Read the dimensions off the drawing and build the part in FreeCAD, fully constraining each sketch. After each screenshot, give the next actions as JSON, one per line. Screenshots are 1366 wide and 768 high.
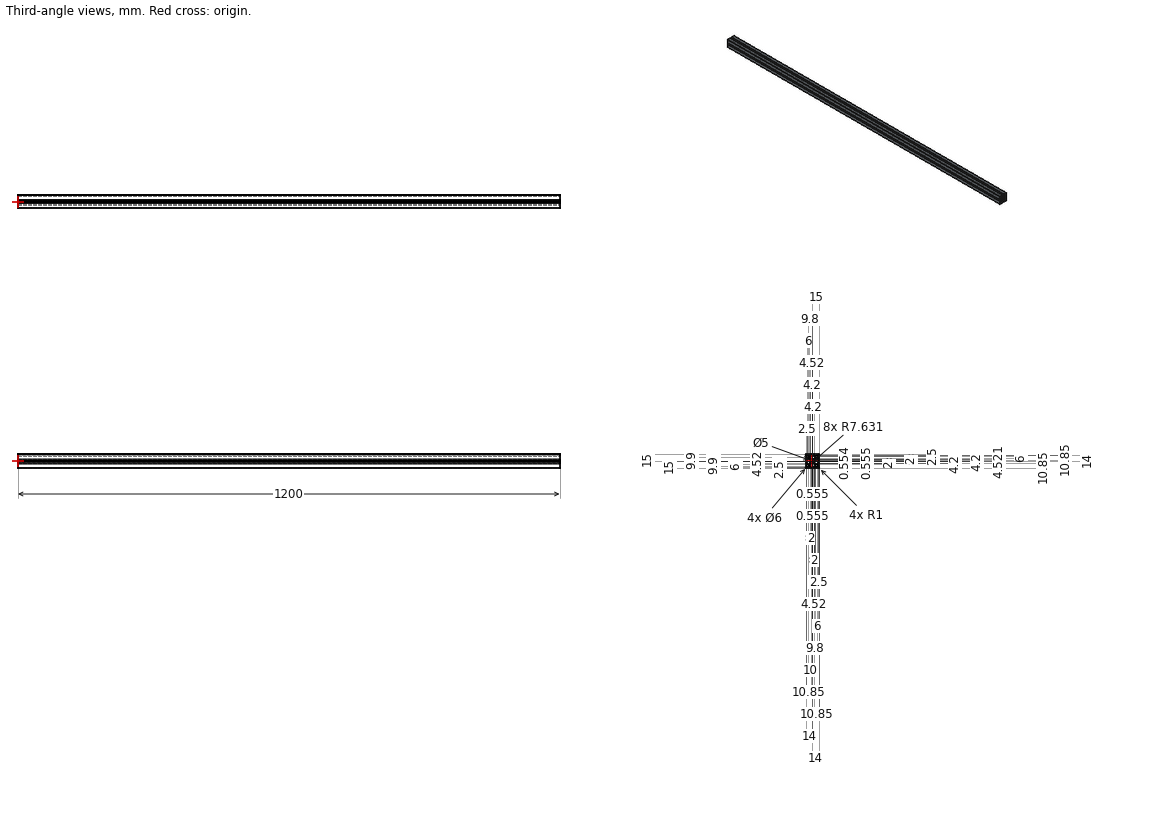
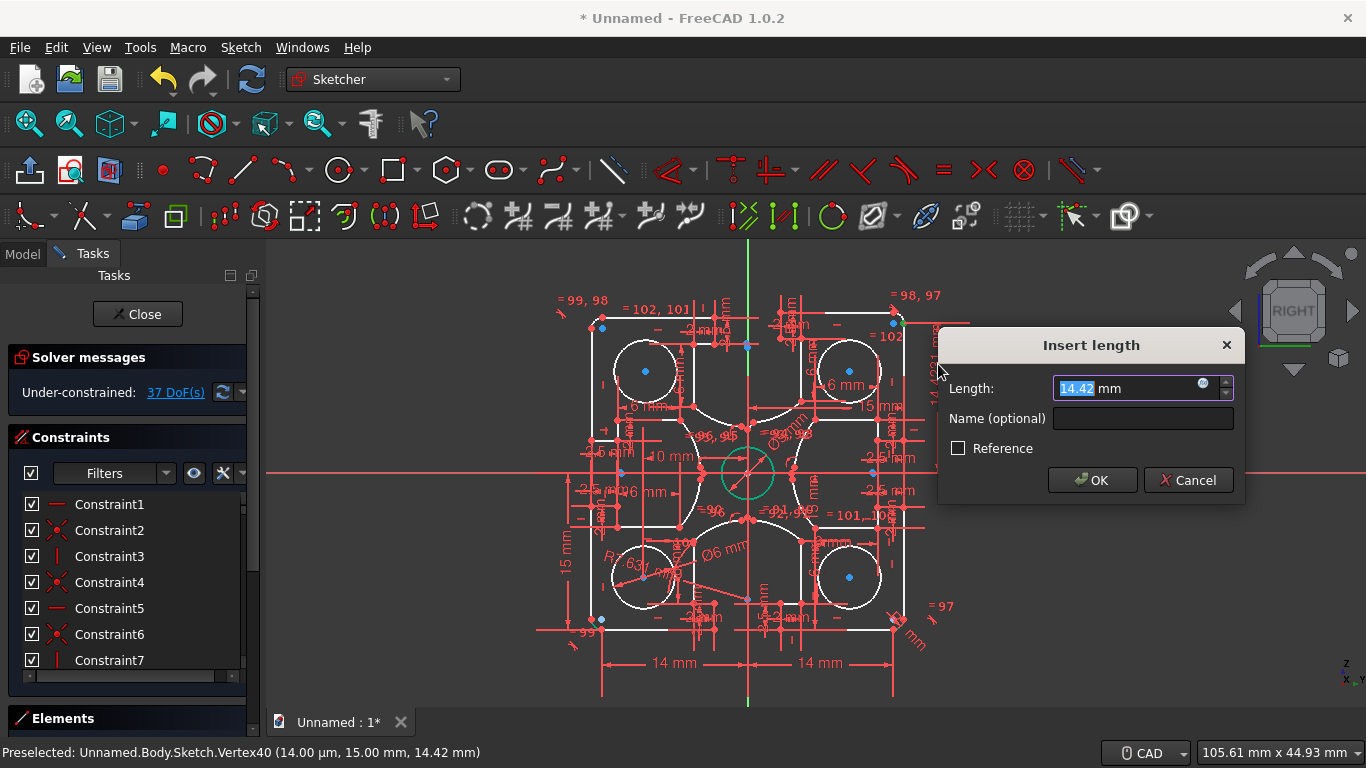
{"action": "type", "text": "14"}
{"action": "key", "text": "Return"}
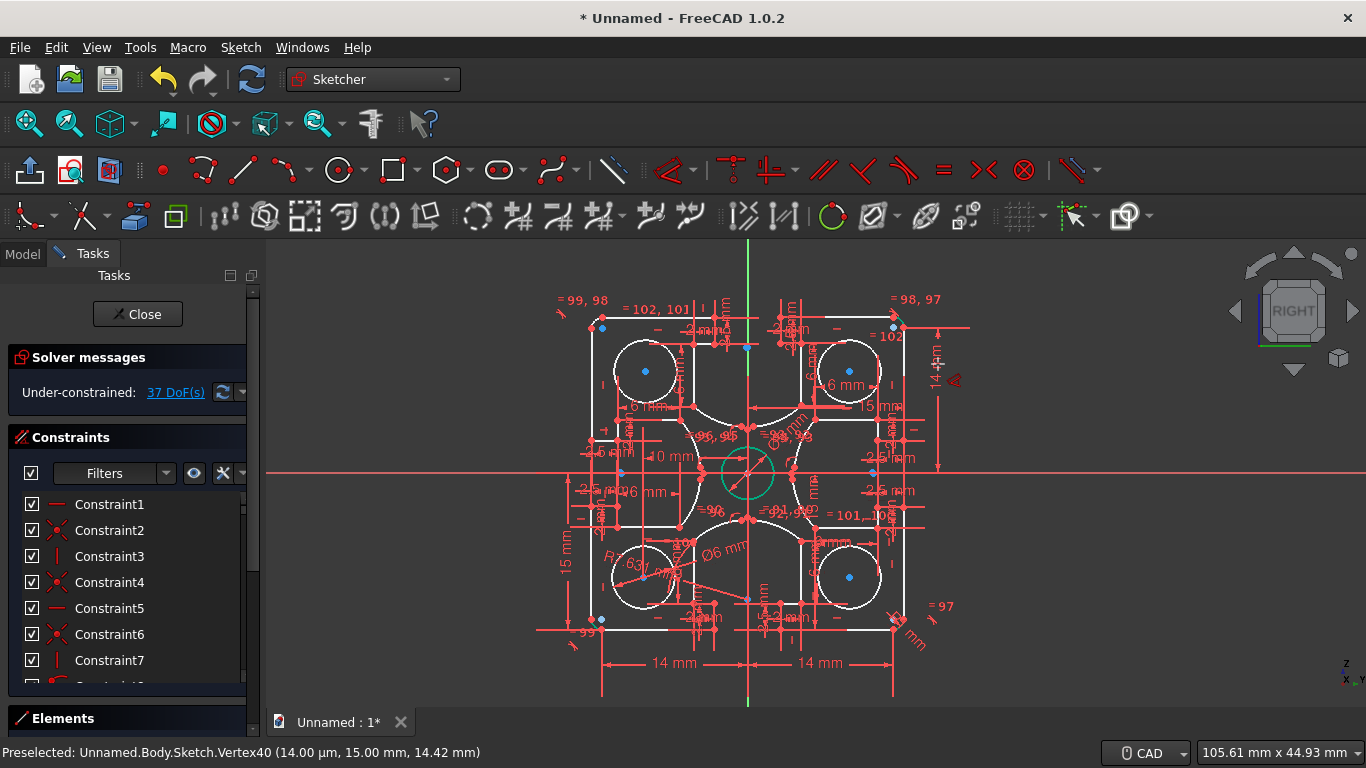
{"action": "left_click", "coordinate": [715, 318]}
{"action": "left_click", "coordinate": [609, 341]}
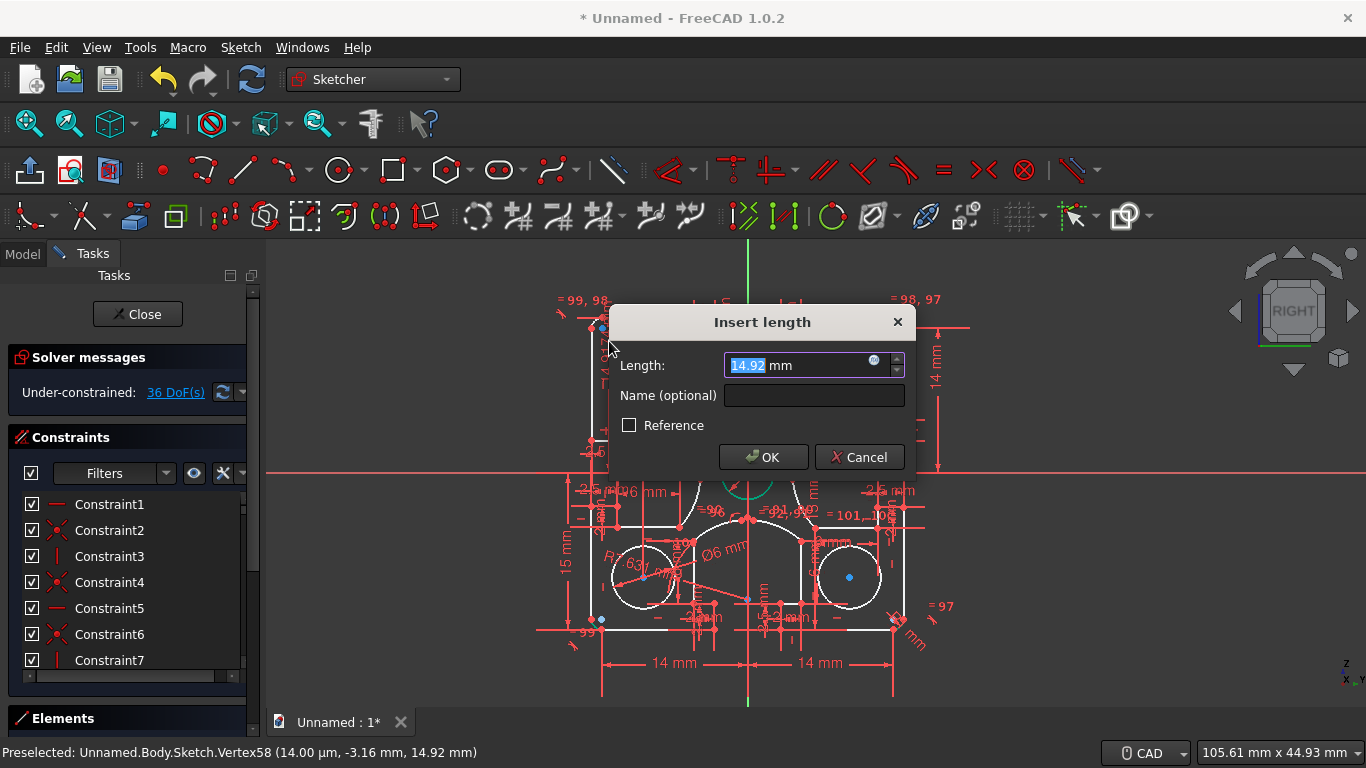
{"action": "type", "text": "15"}
{"action": "key", "text": "Return"}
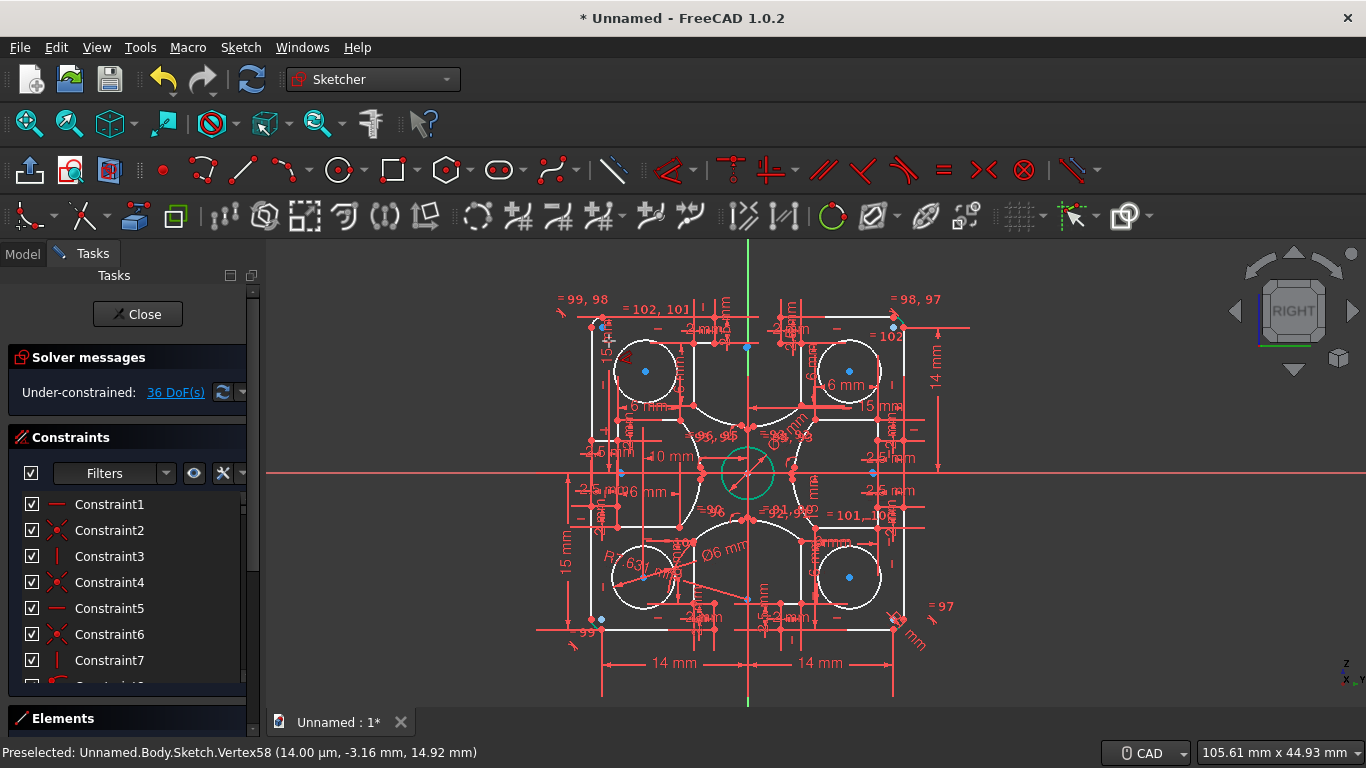
{"action": "left_click", "coordinate": [602, 317]}
{"action": "left_click", "coordinate": [675, 283]}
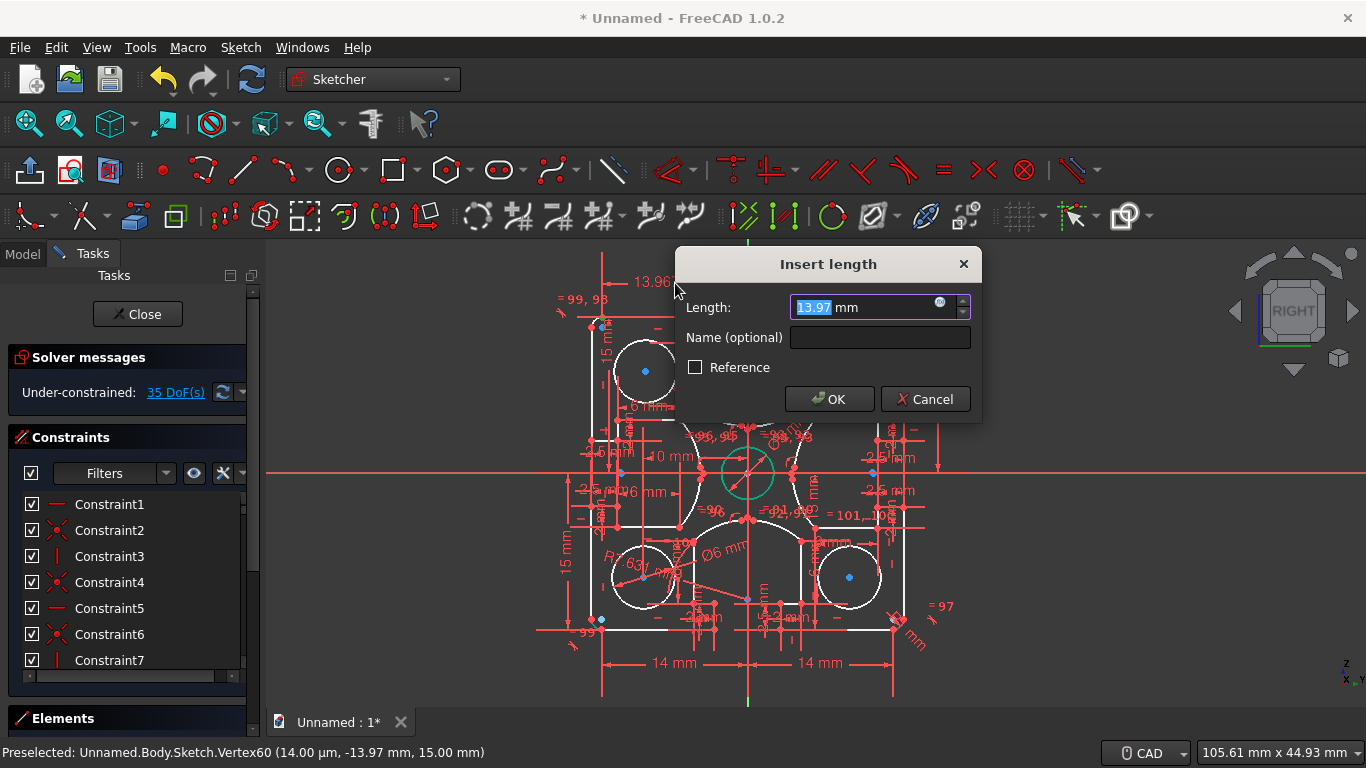
{"action": "type", "text": "14"}
{"action": "key", "text": "Return"}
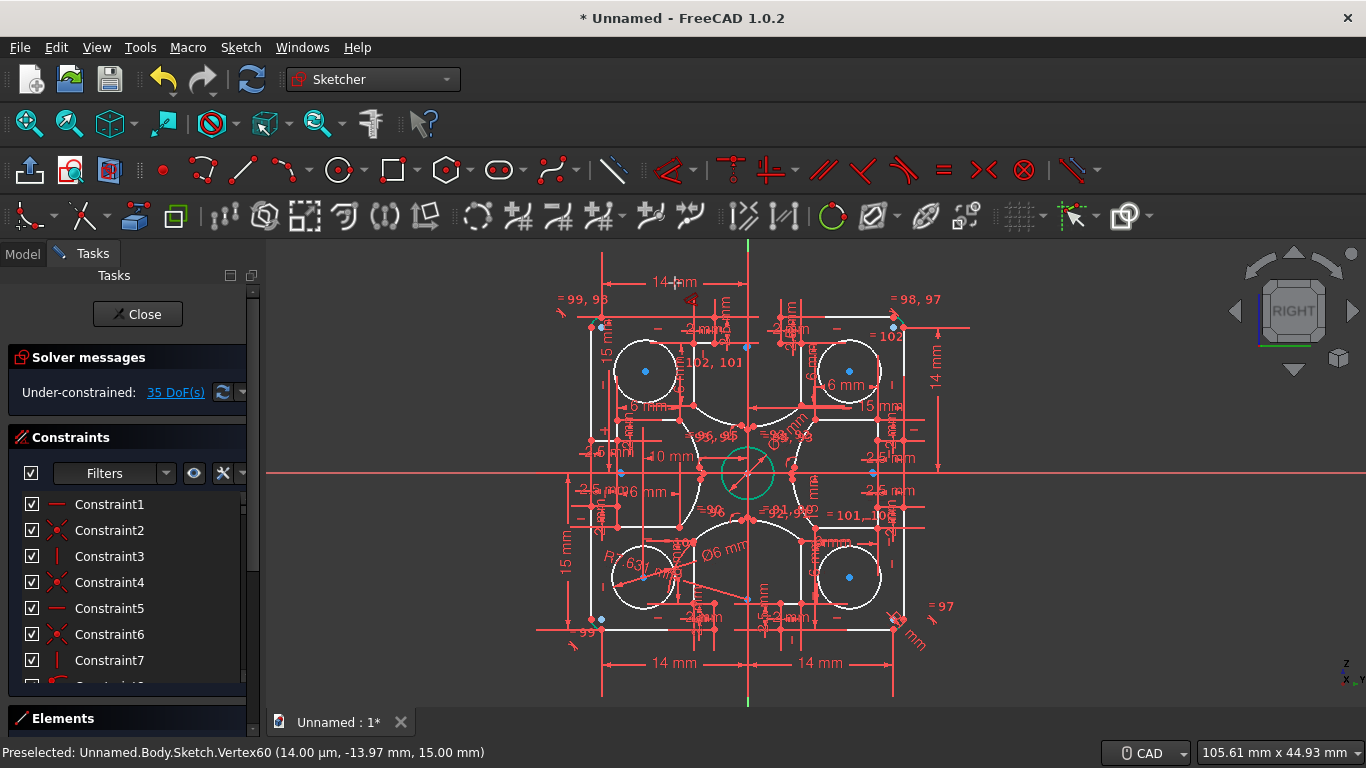
{"action": "left_click", "coordinate": [643, 578]}
{"action": "left_click", "coordinate": [513, 525]}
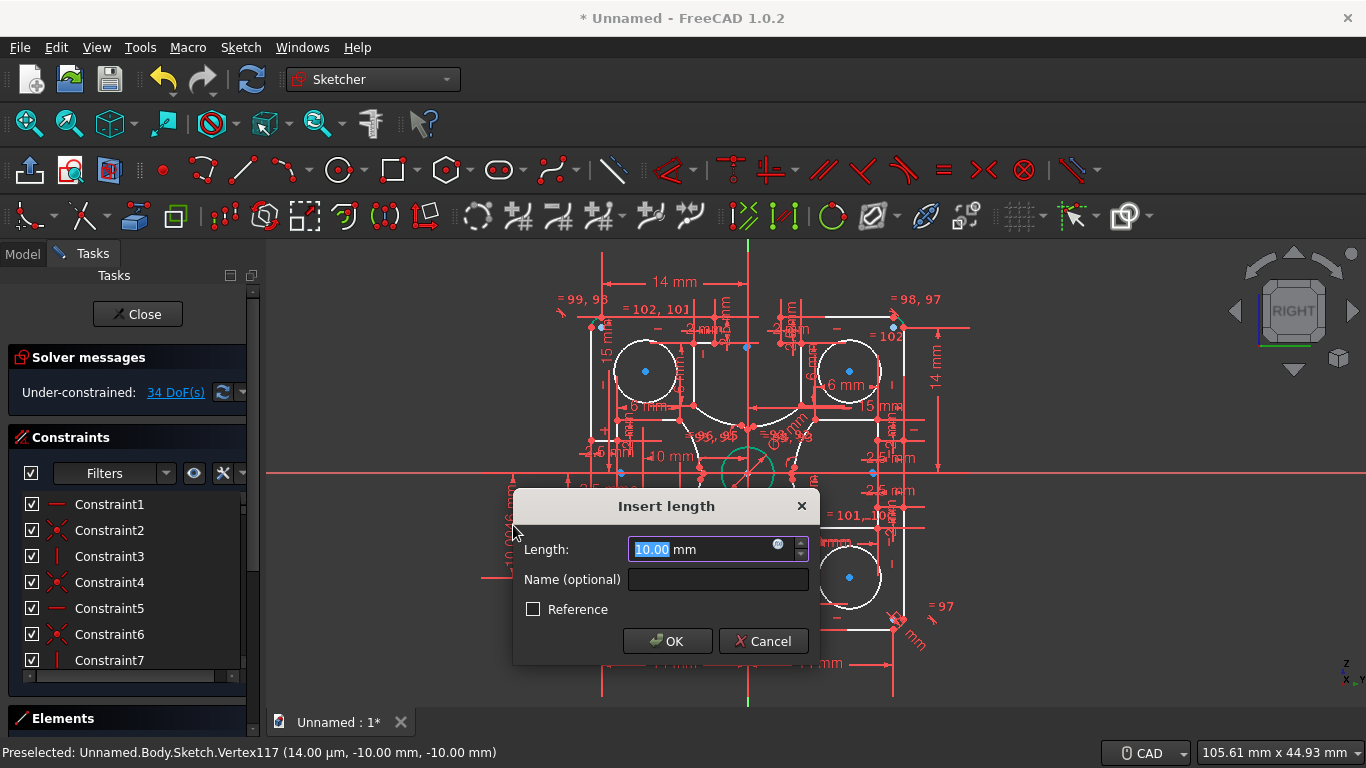
{"action": "type", "text": "9.9"}
{"action": "key", "text": "Return"}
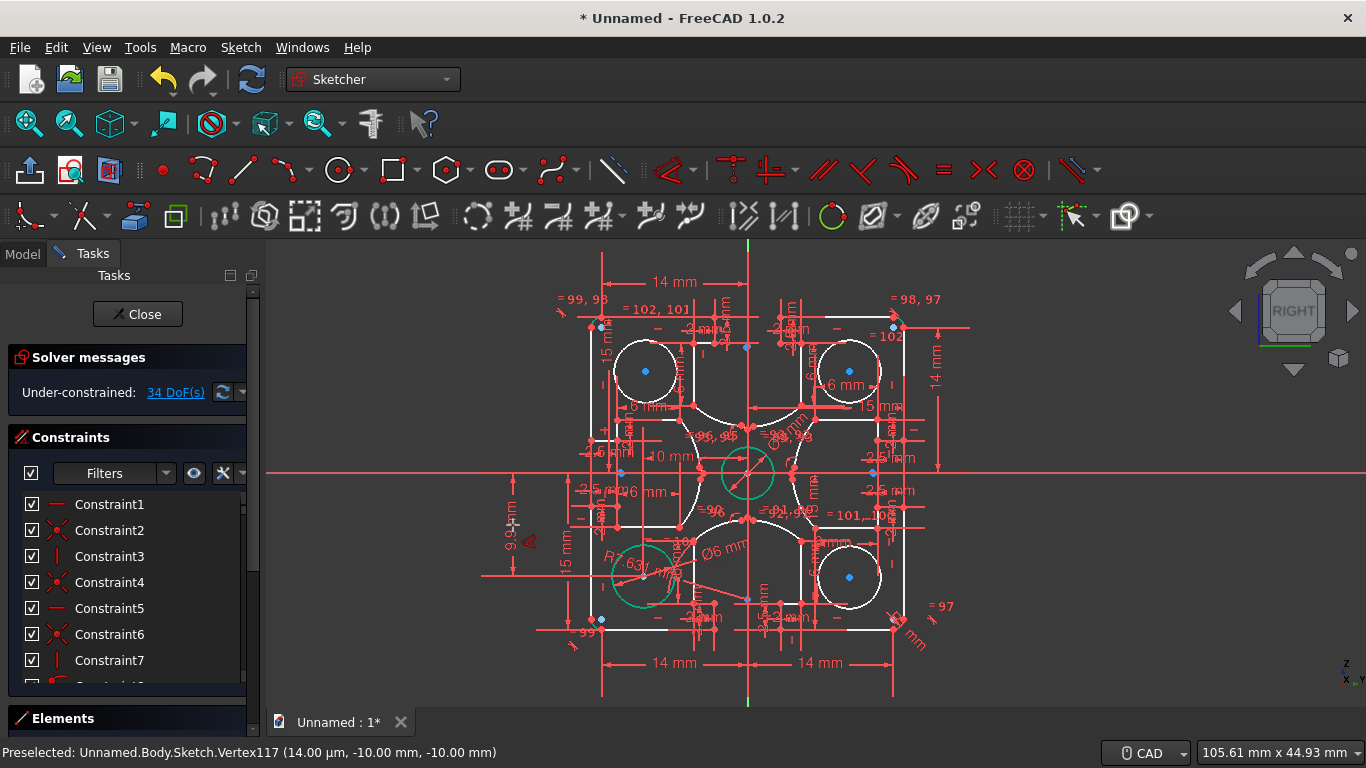
{"action": "left_click", "coordinate": [850, 578]}
{"action": "left_click", "coordinate": [775, 391]}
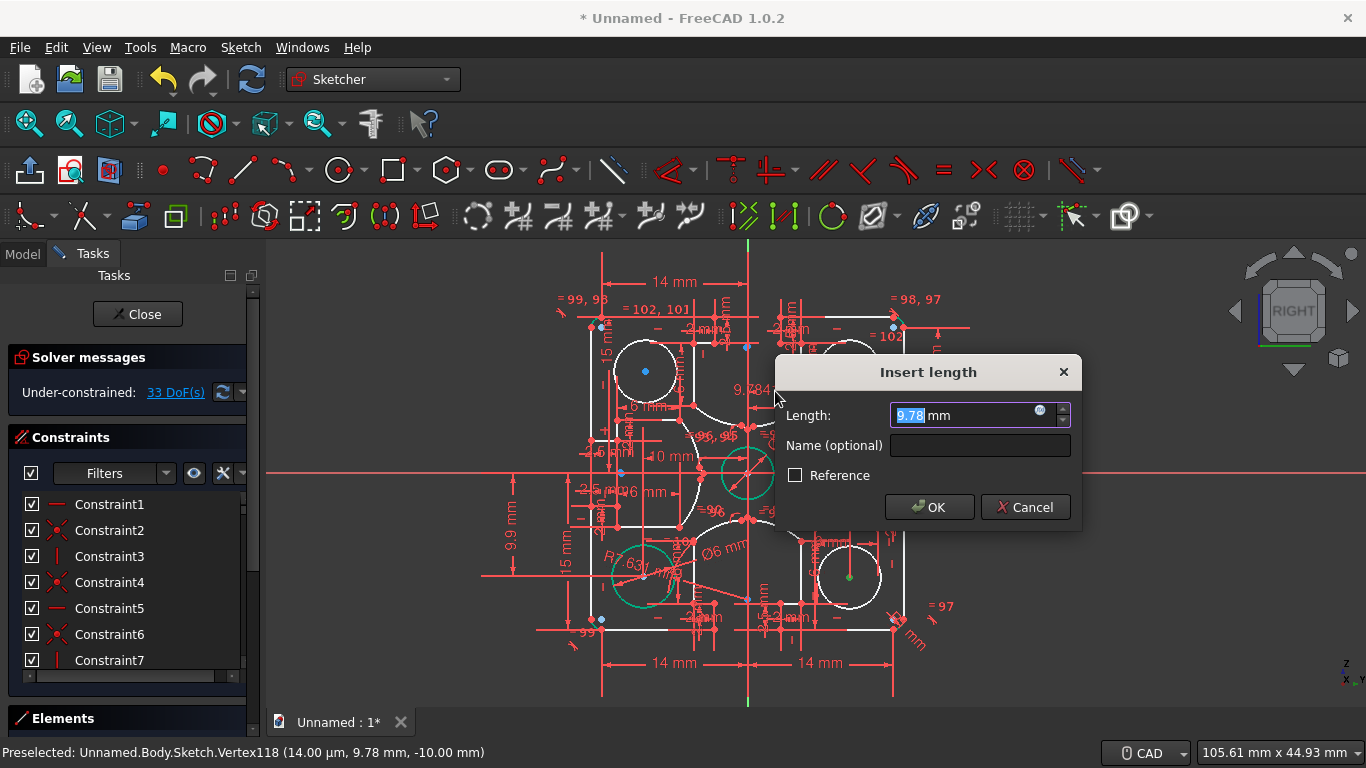
{"action": "type", "text": "9.8"}
{"action": "key", "text": "Return"}